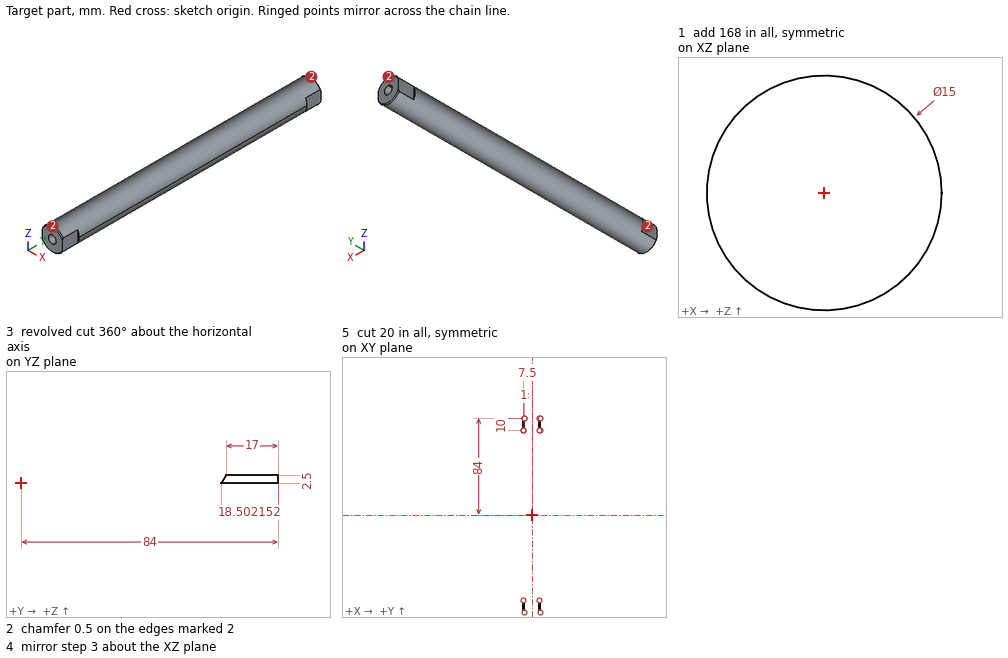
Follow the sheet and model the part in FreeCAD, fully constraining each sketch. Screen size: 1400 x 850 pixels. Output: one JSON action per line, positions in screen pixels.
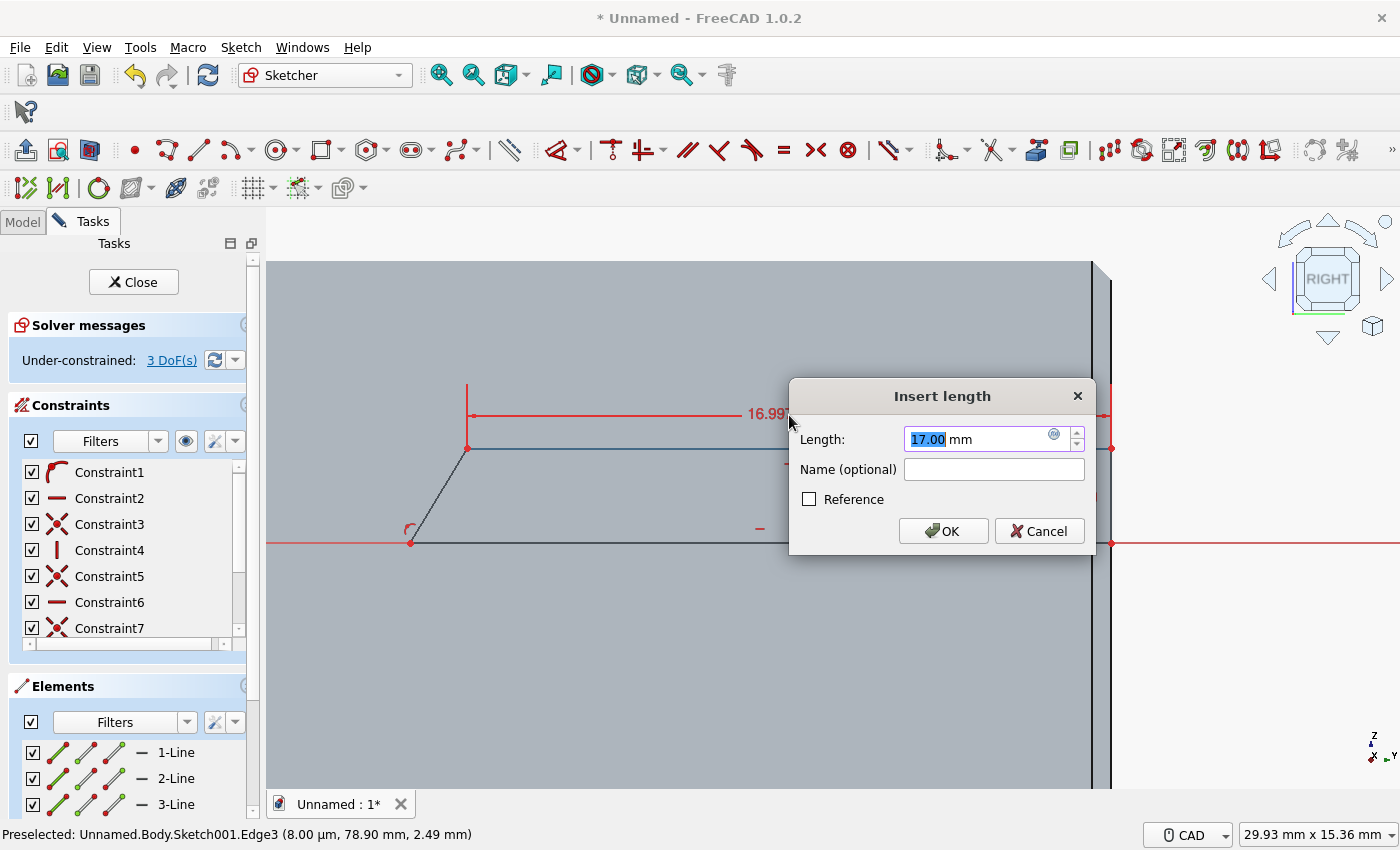
{"action": "type", "text": "17"}
{"action": "key", "text": "Return"}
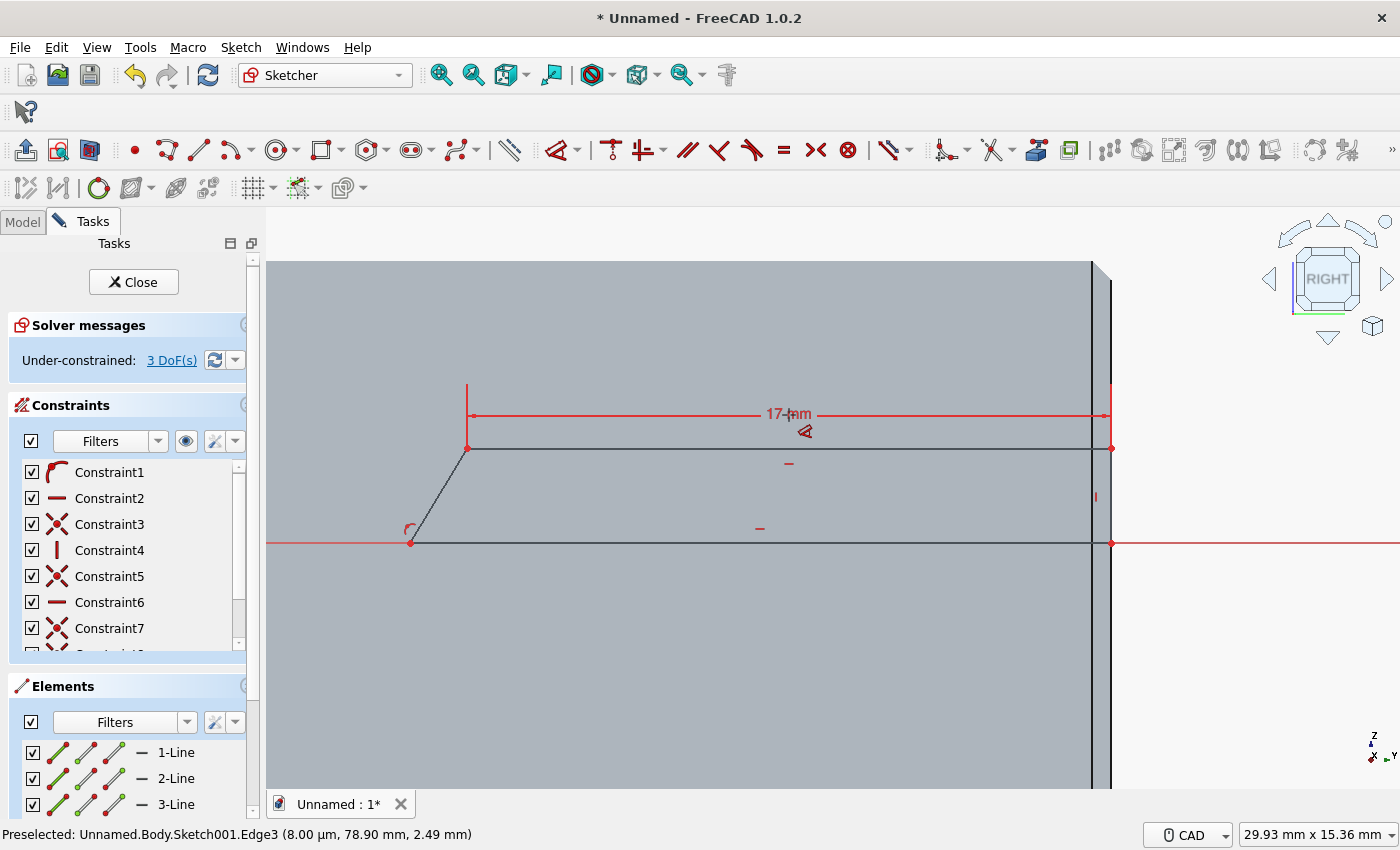
{"action": "left_click", "coordinate": [1111, 515]}
{"action": "left_click", "coordinate": [1145, 496]}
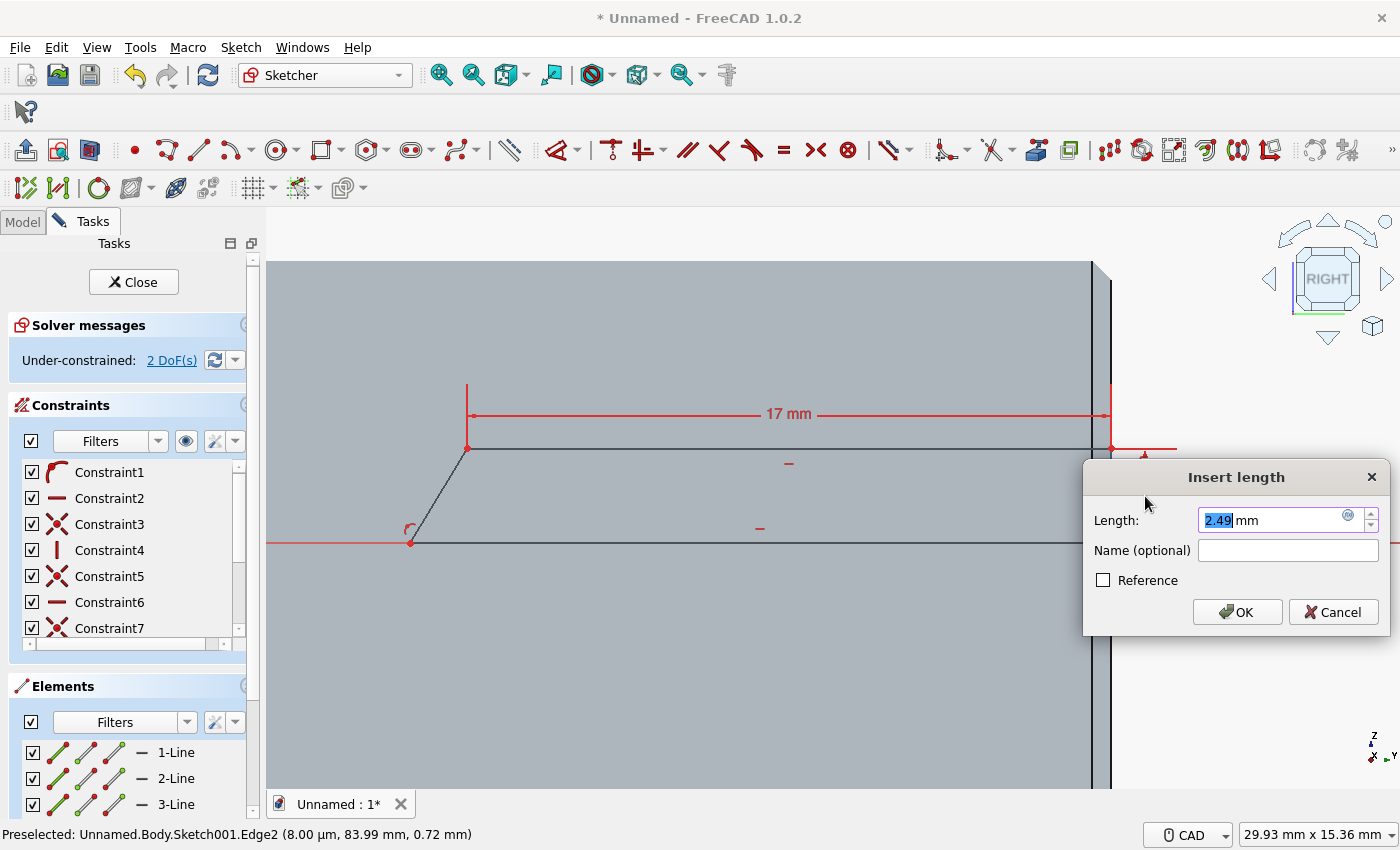
{"action": "type", "text": "2.5"}
{"action": "key", "text": "Return"}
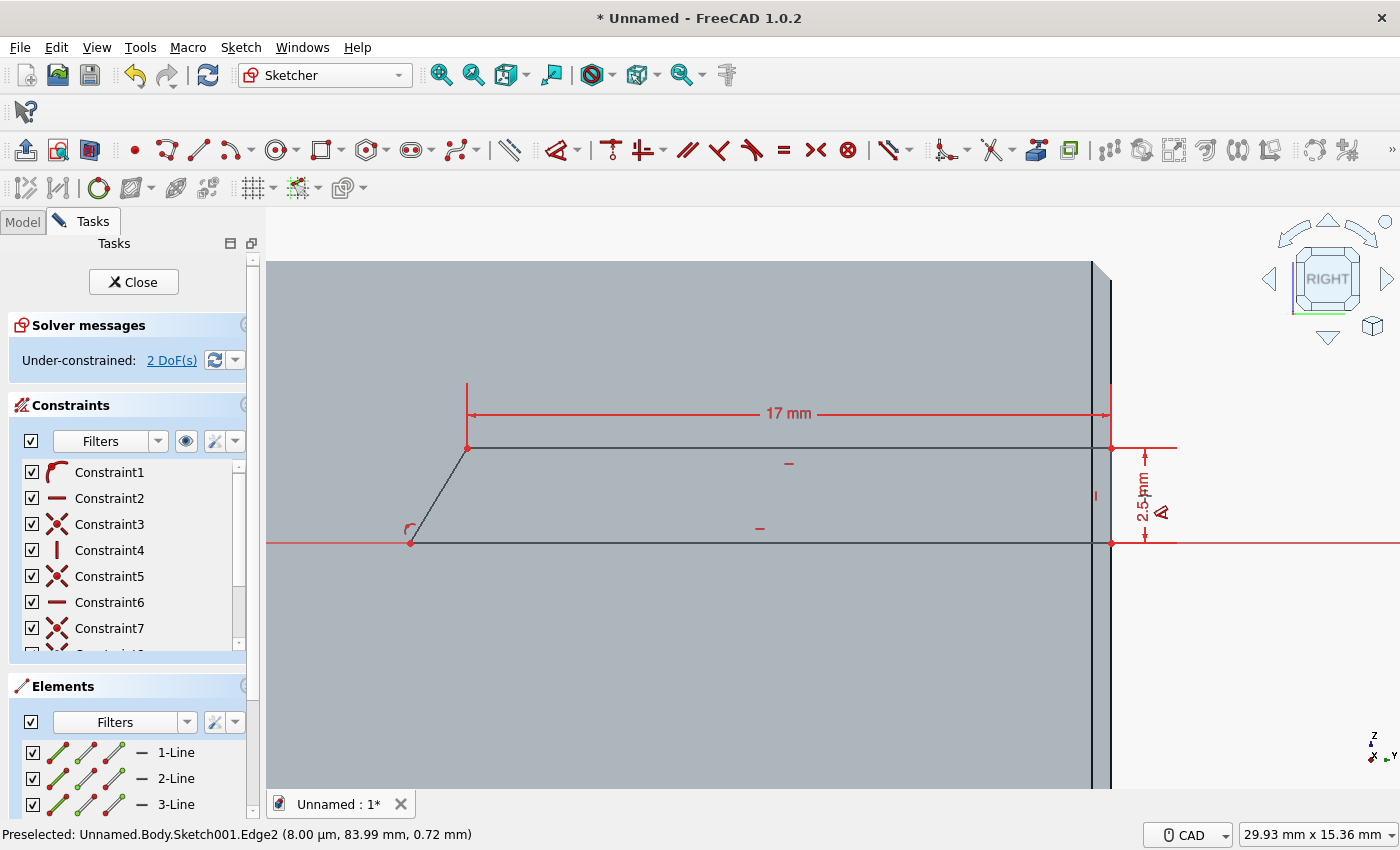
{"action": "left_click", "coordinate": [1111, 543]}
{"action": "left_click", "coordinate": [703, 577]}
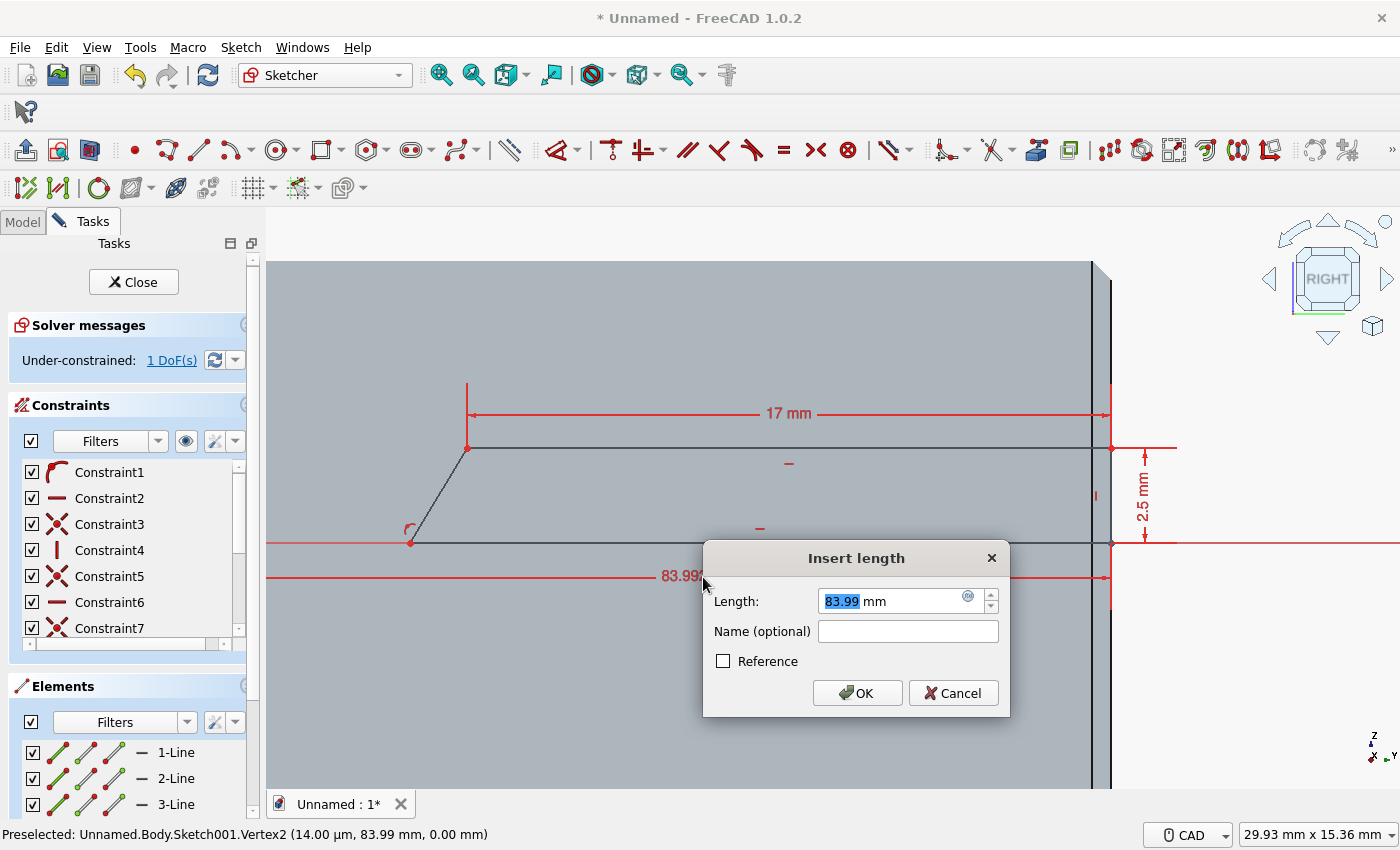
{"action": "type", "text": "84"}
{"action": "key", "text": "Return"}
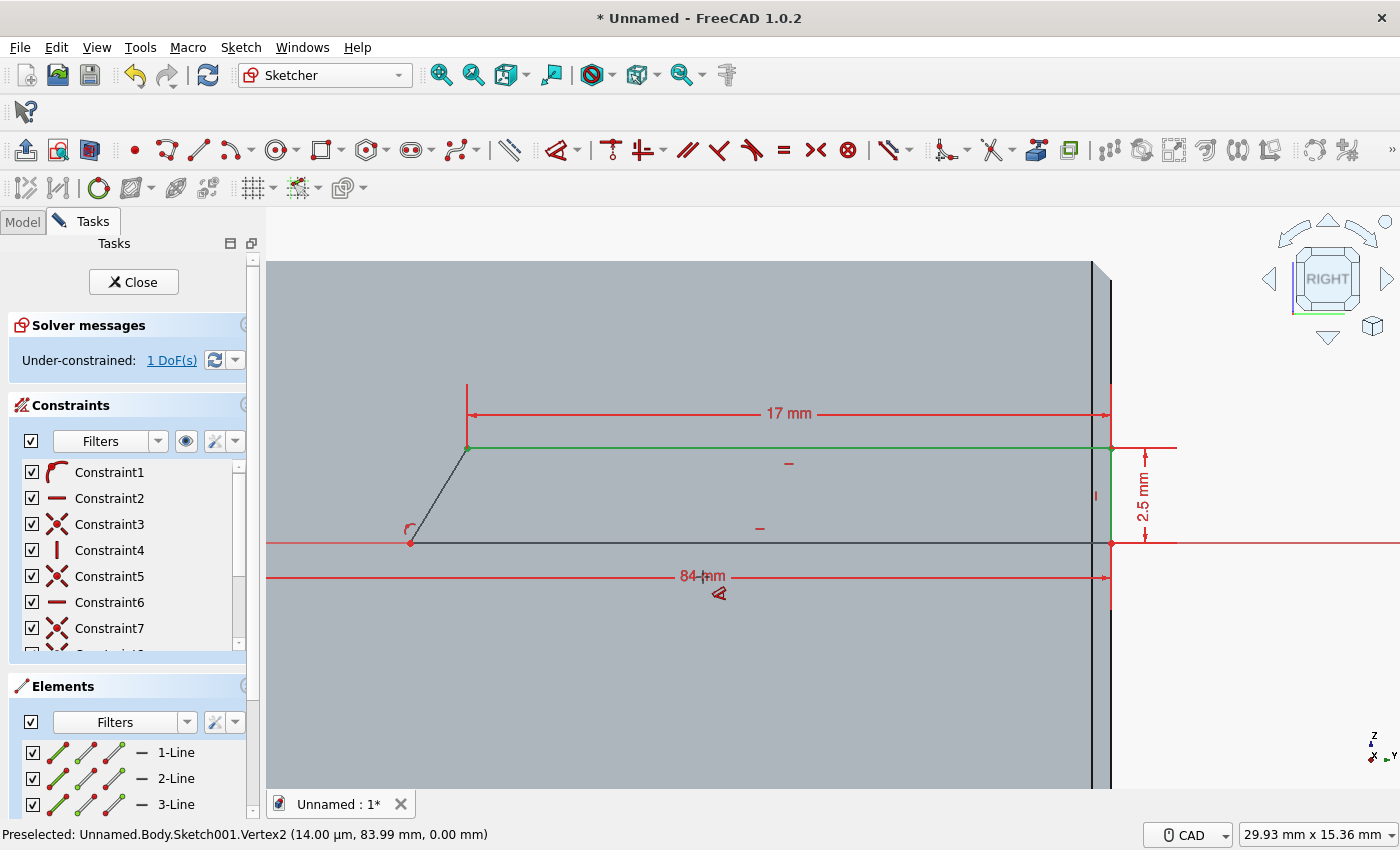
{"action": "left_click", "coordinate": [620, 543]}
{"action": "left_click", "coordinate": [599, 577]}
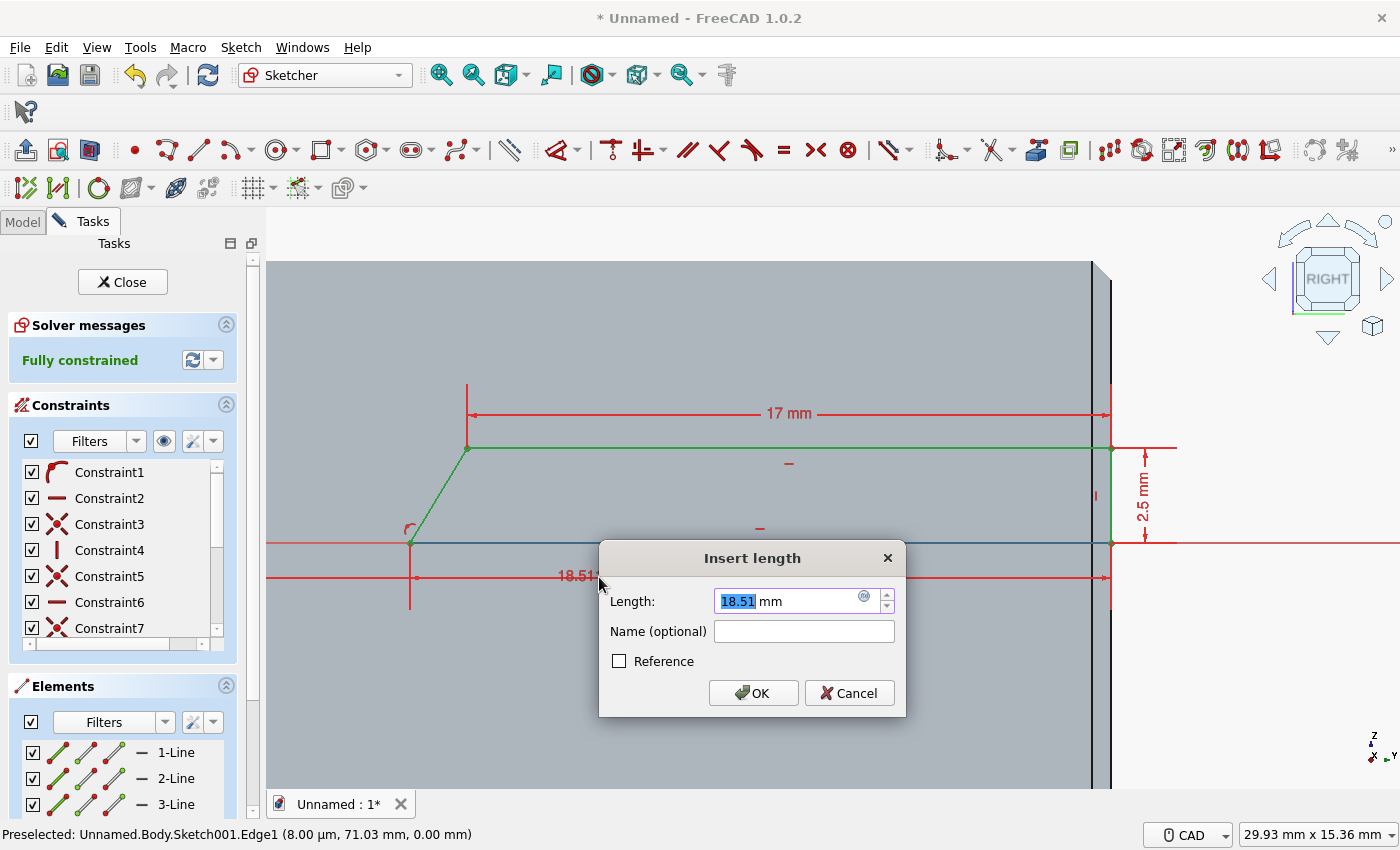
{"action": "type", "text": "18.502152"}
{"action": "key", "text": "Return"}
{"action": "key", "text": "Escape"}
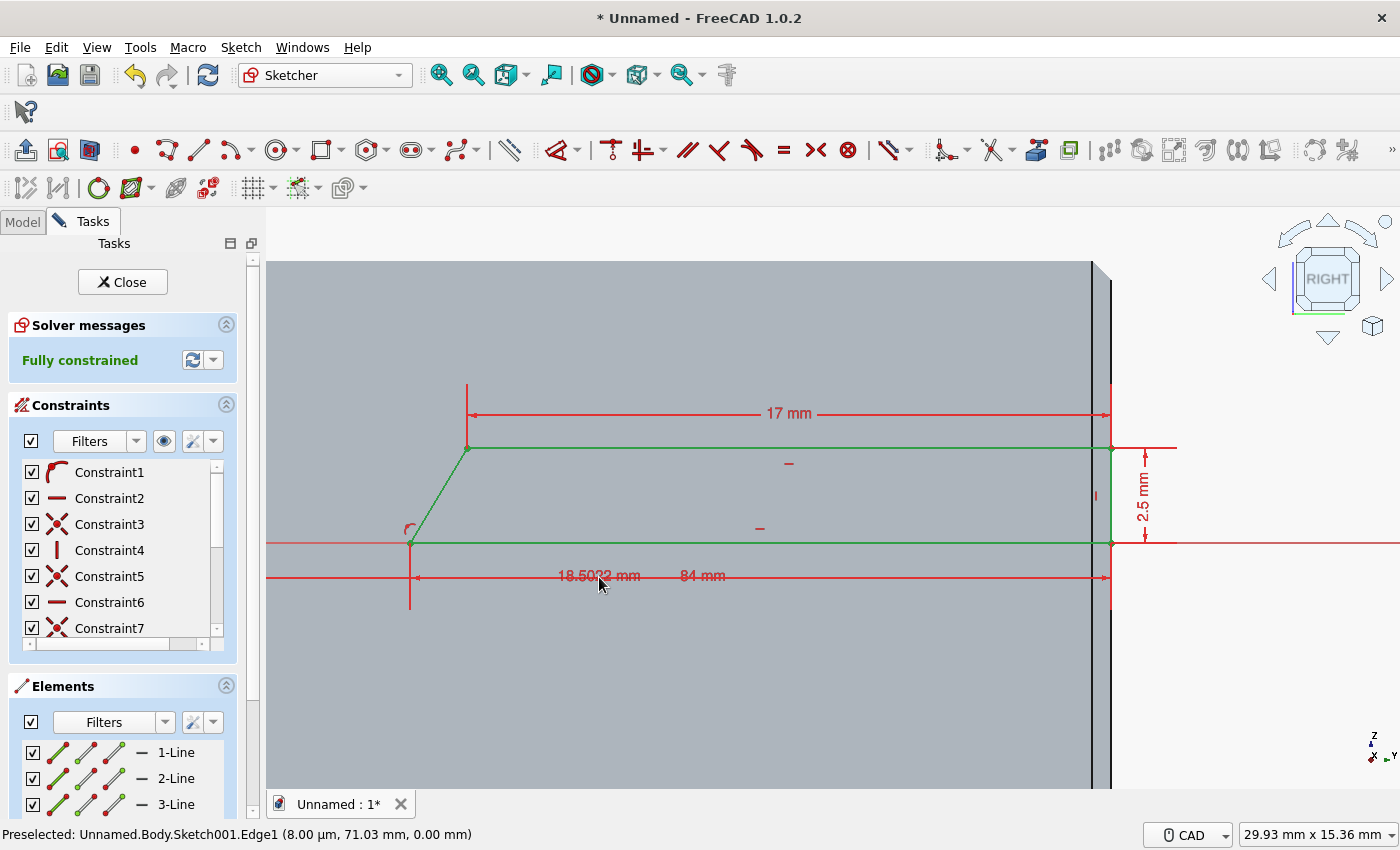
{"action": "left_click", "coordinate": [123, 282]}